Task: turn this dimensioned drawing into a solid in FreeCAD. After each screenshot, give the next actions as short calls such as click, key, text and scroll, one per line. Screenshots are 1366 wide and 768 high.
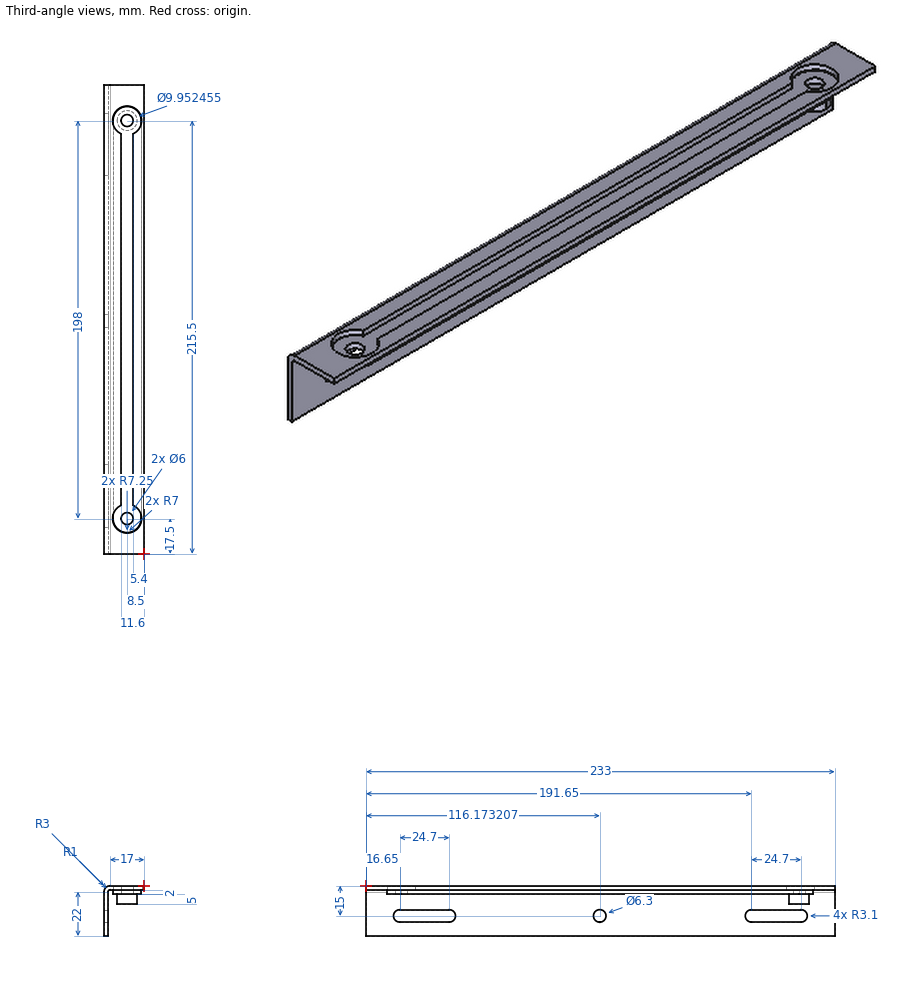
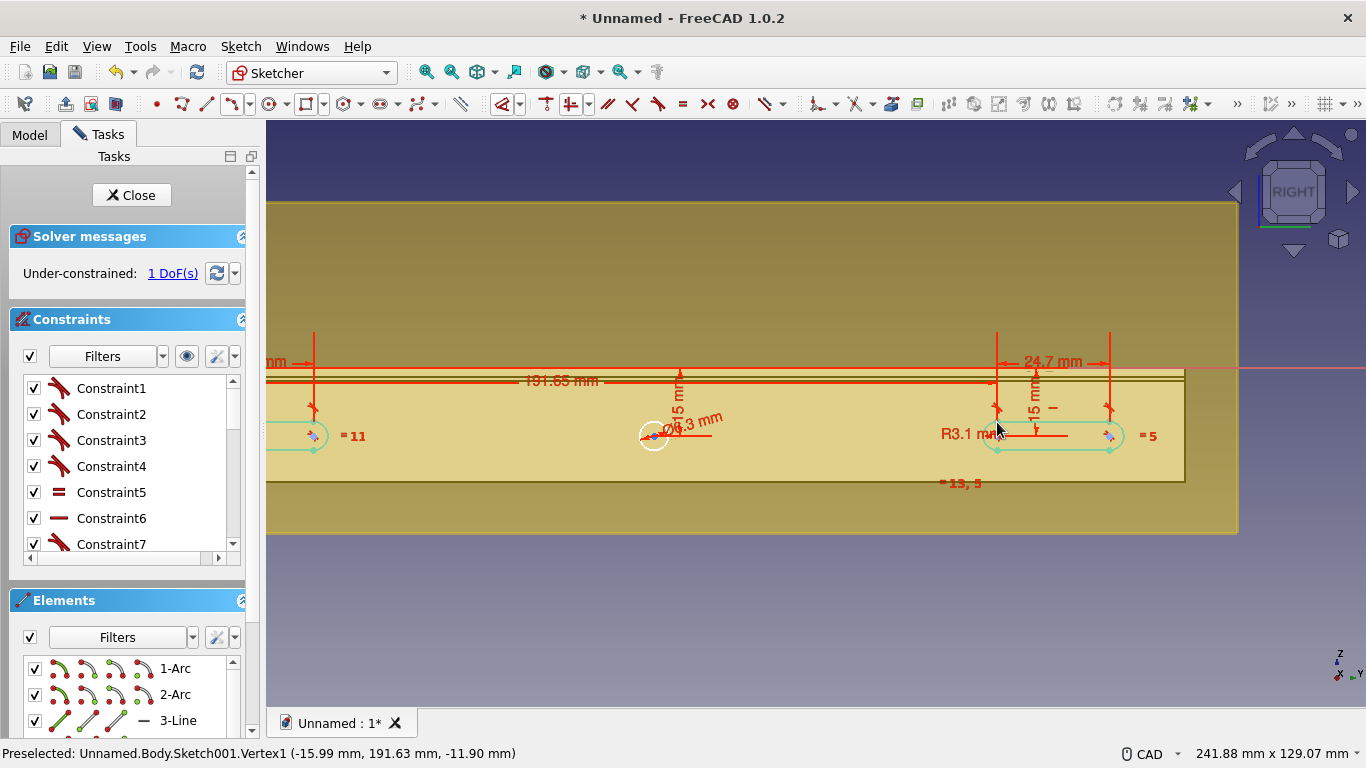
click(654, 436)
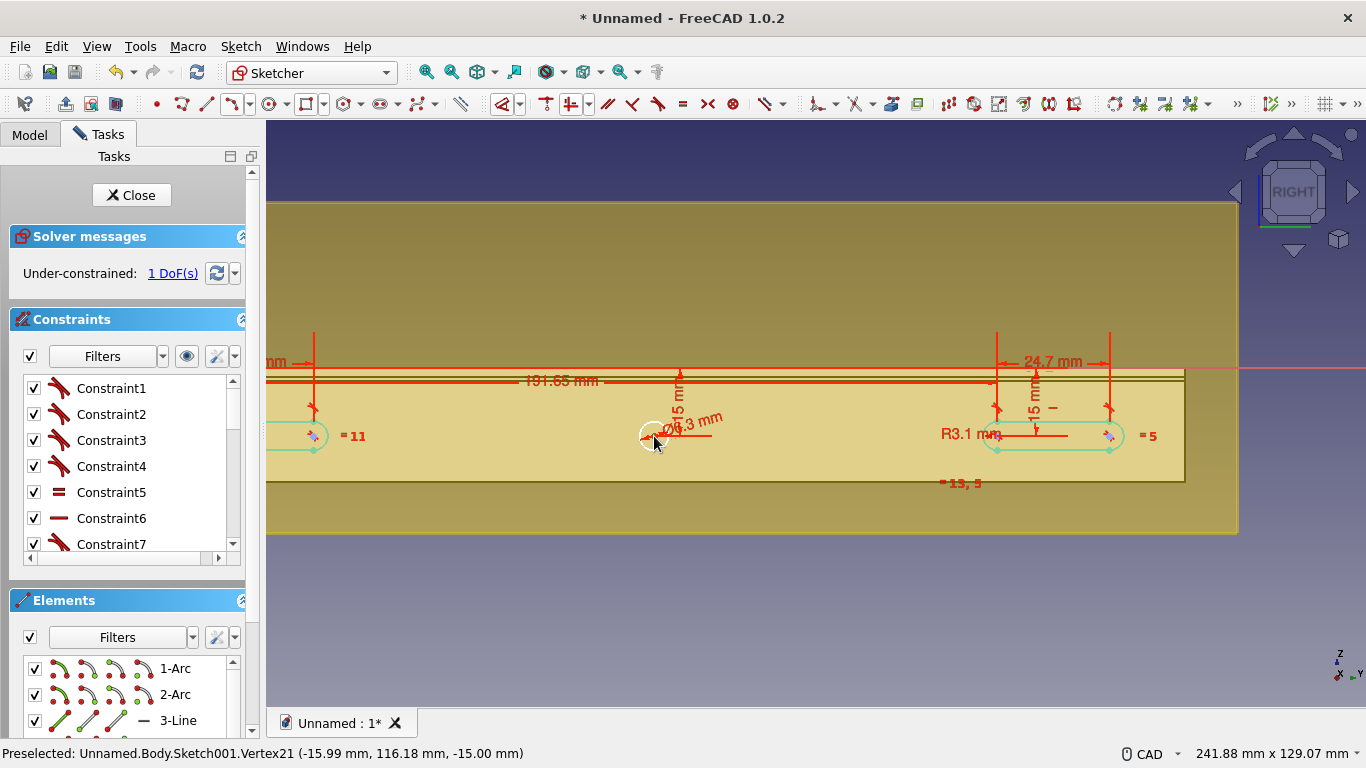
click(520, 104)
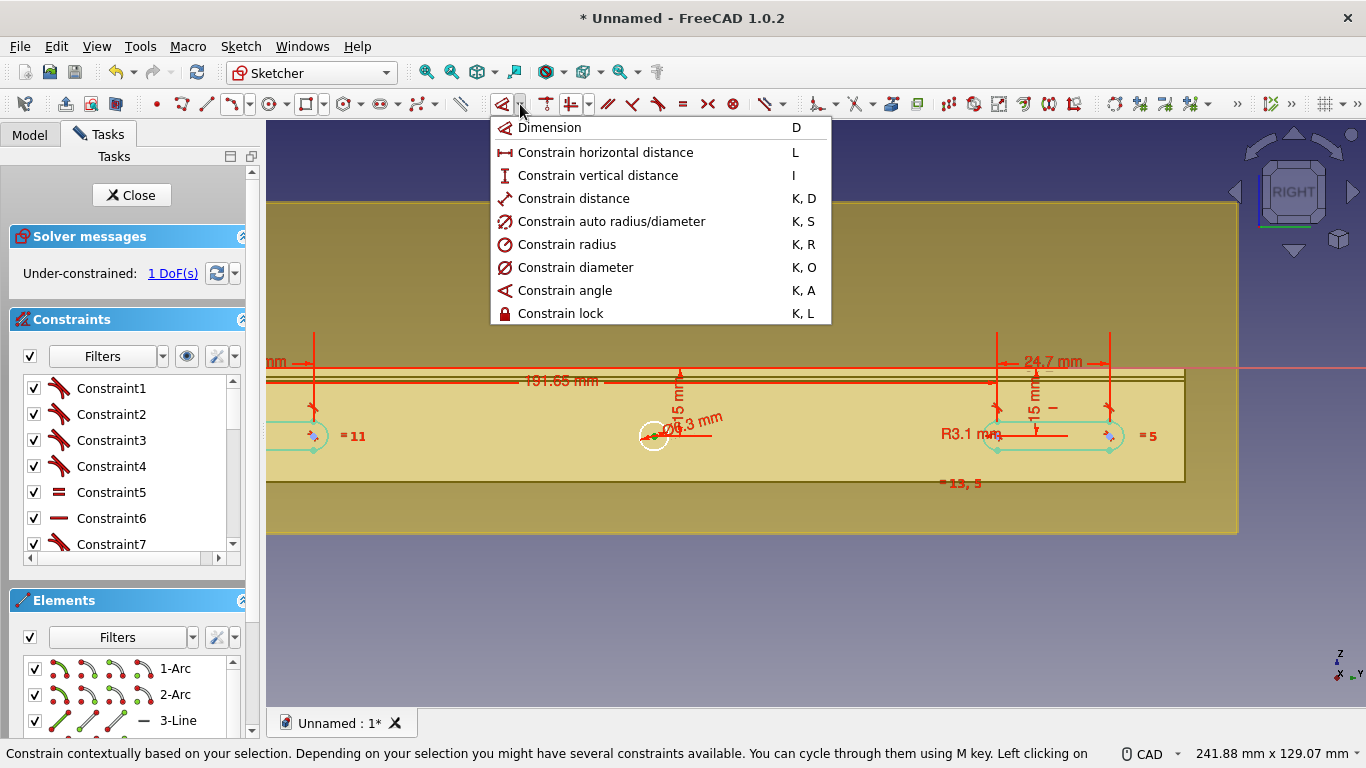
click(661, 152)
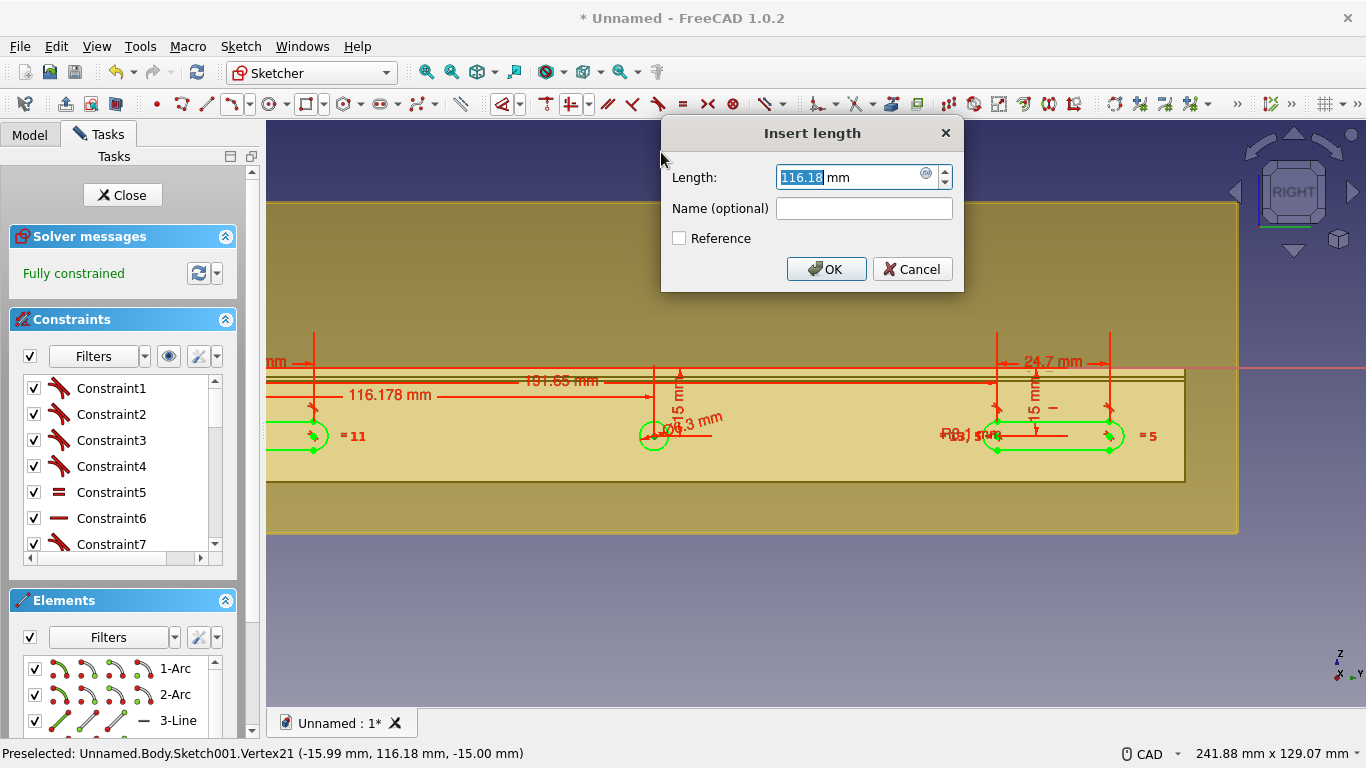
text(116.173207)
key(Return)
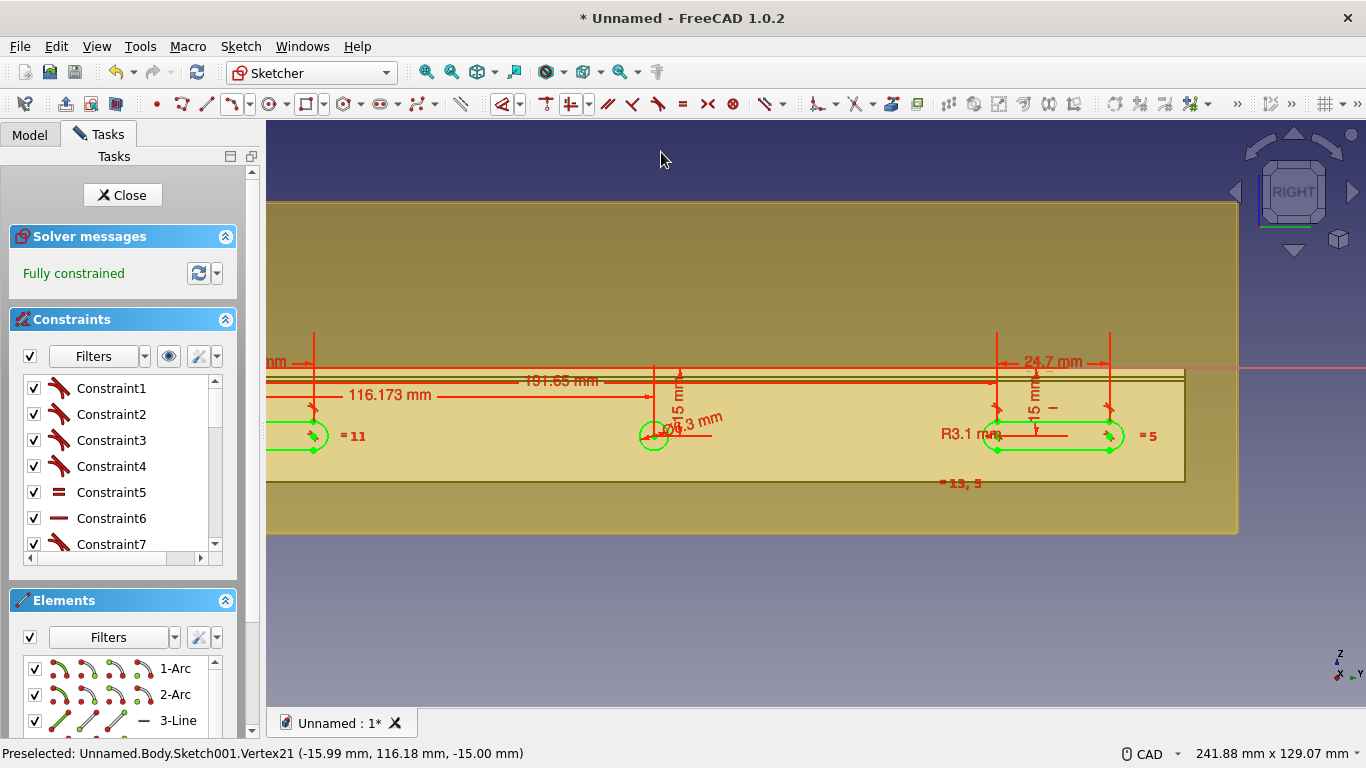
click(123, 195)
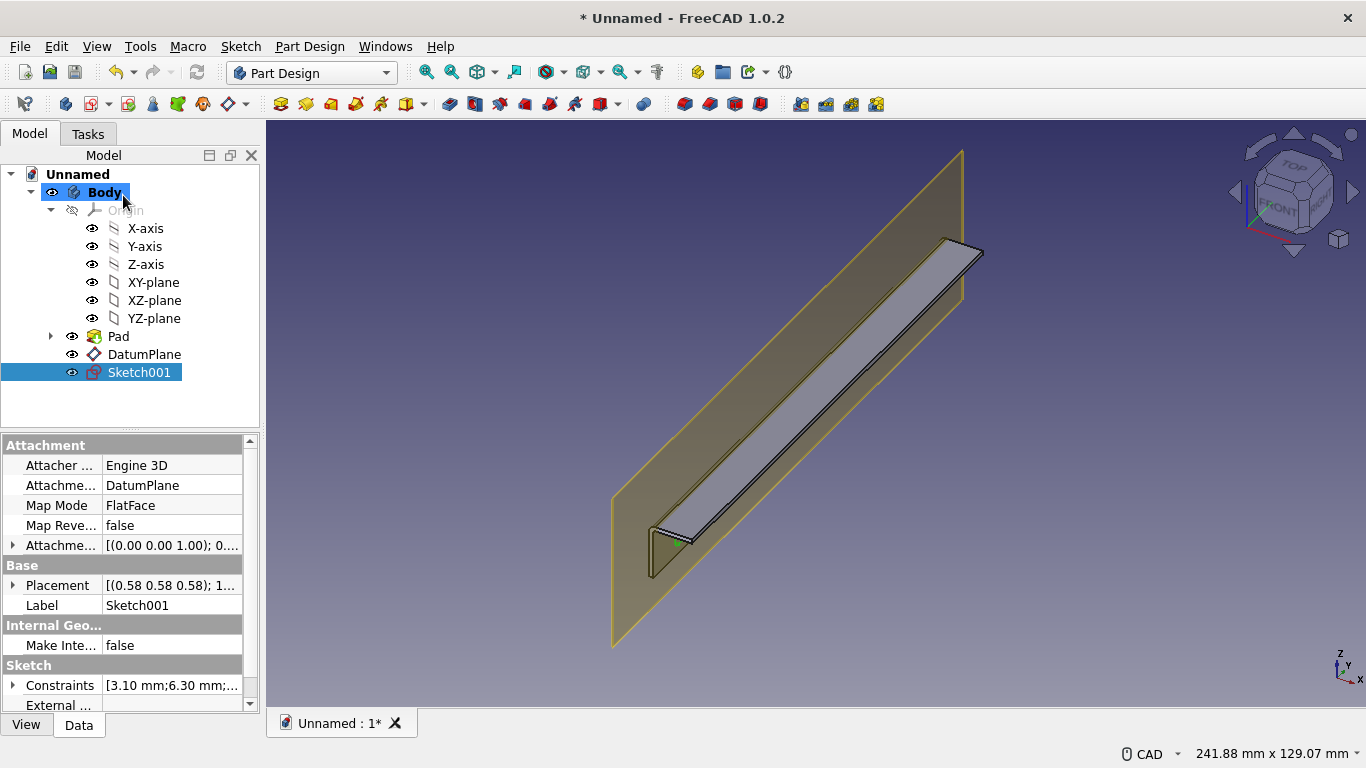
click(450, 104)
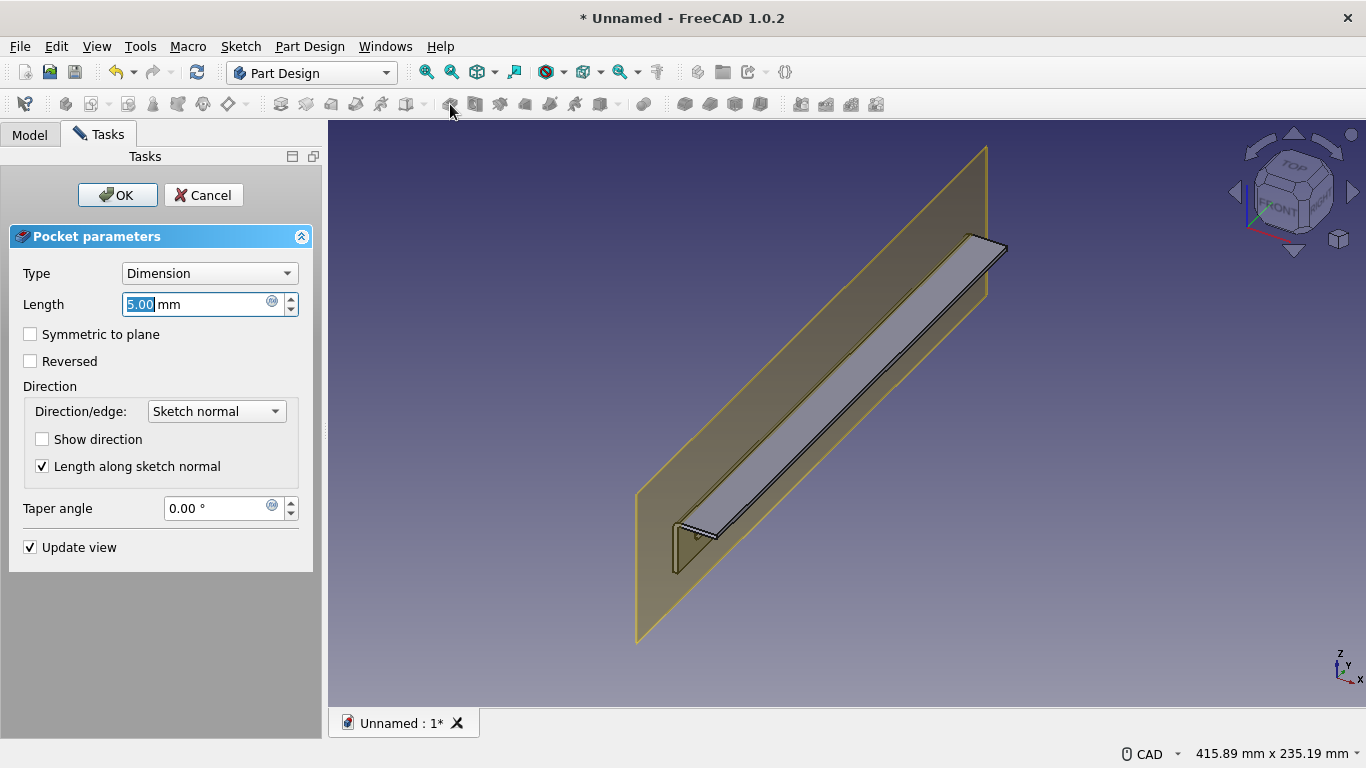
click(210, 274)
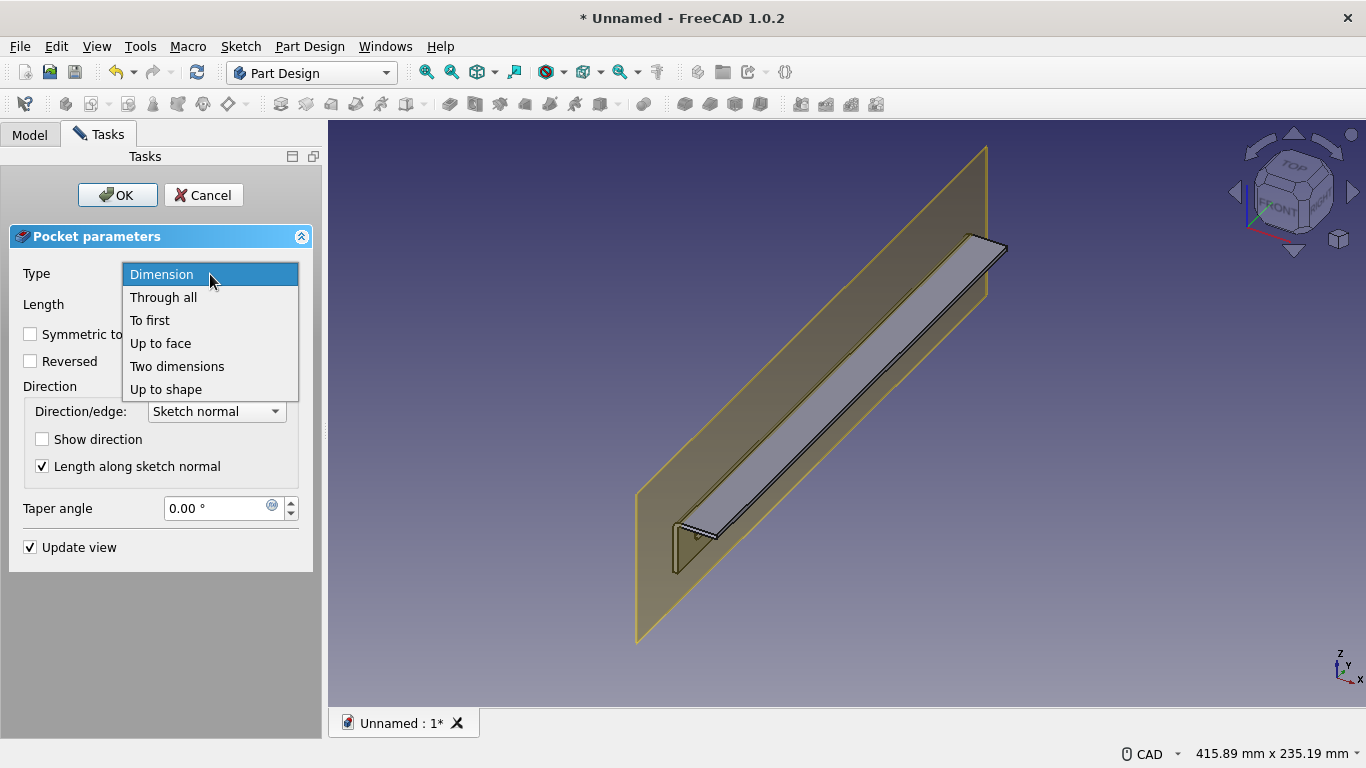
click(208, 298)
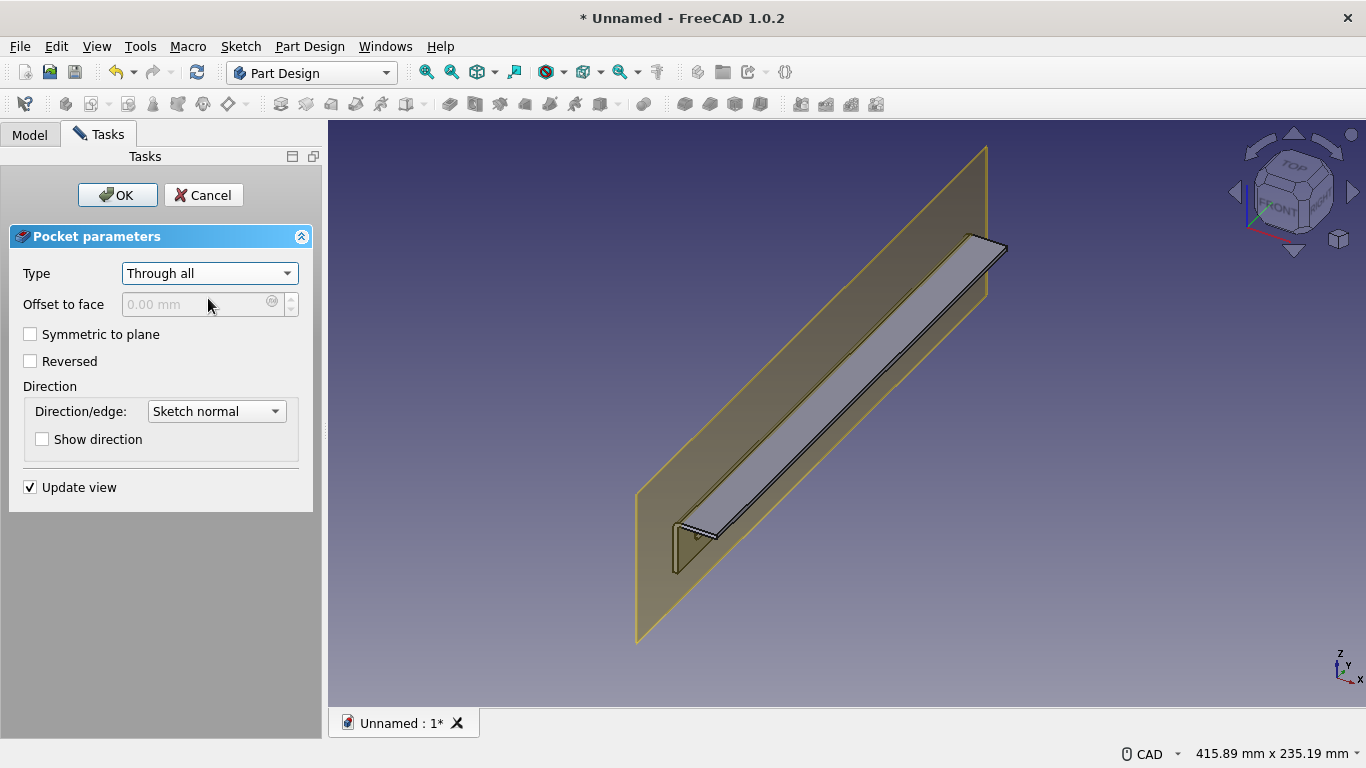
click(118, 195)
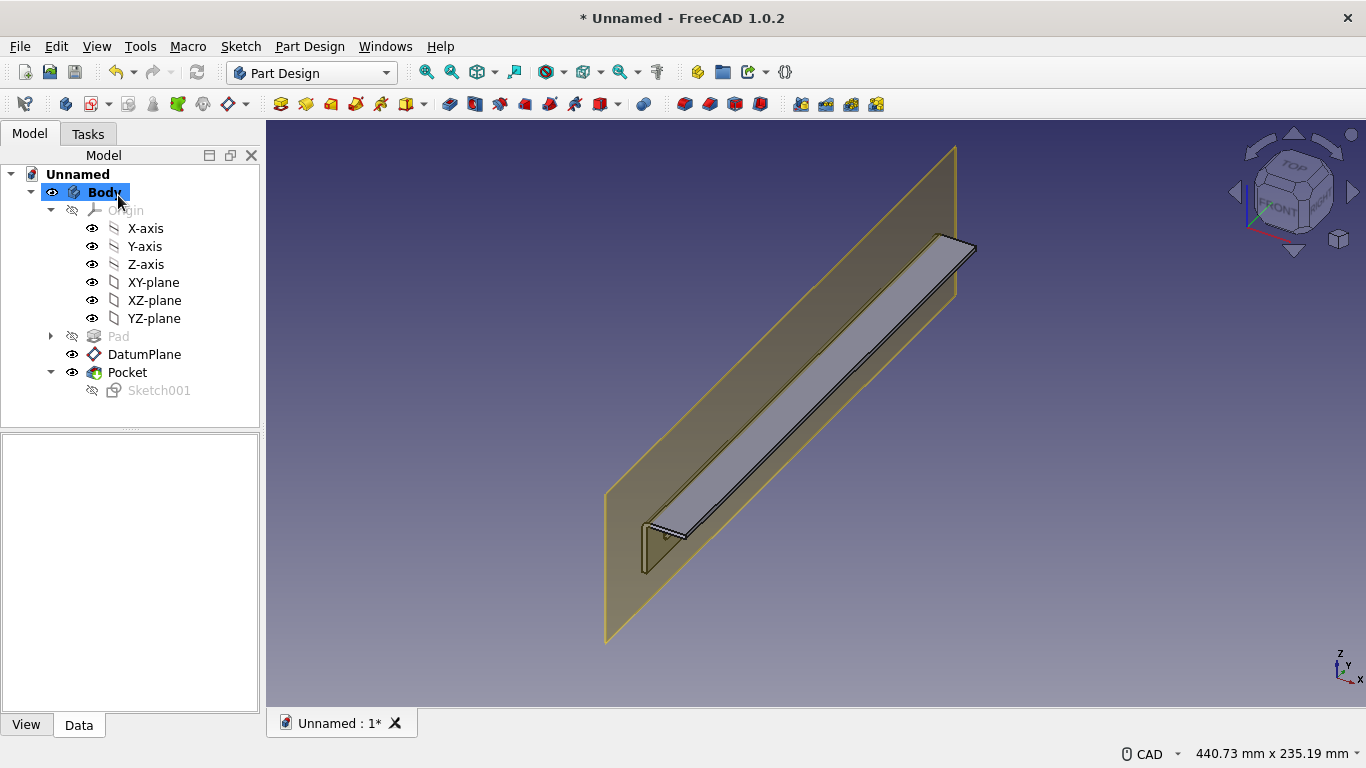
click(117, 354)
key(space)